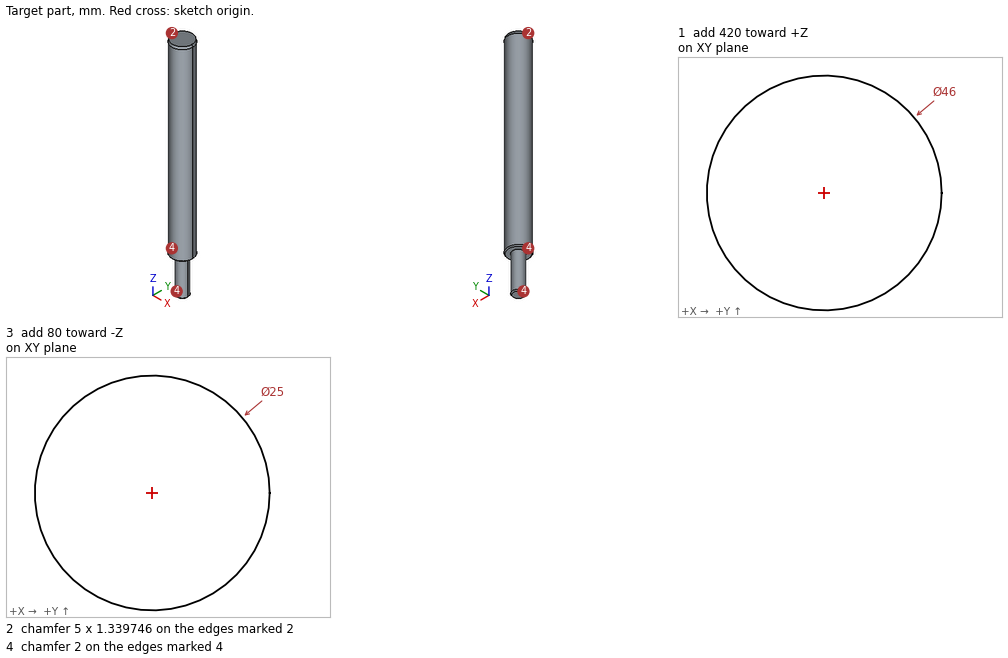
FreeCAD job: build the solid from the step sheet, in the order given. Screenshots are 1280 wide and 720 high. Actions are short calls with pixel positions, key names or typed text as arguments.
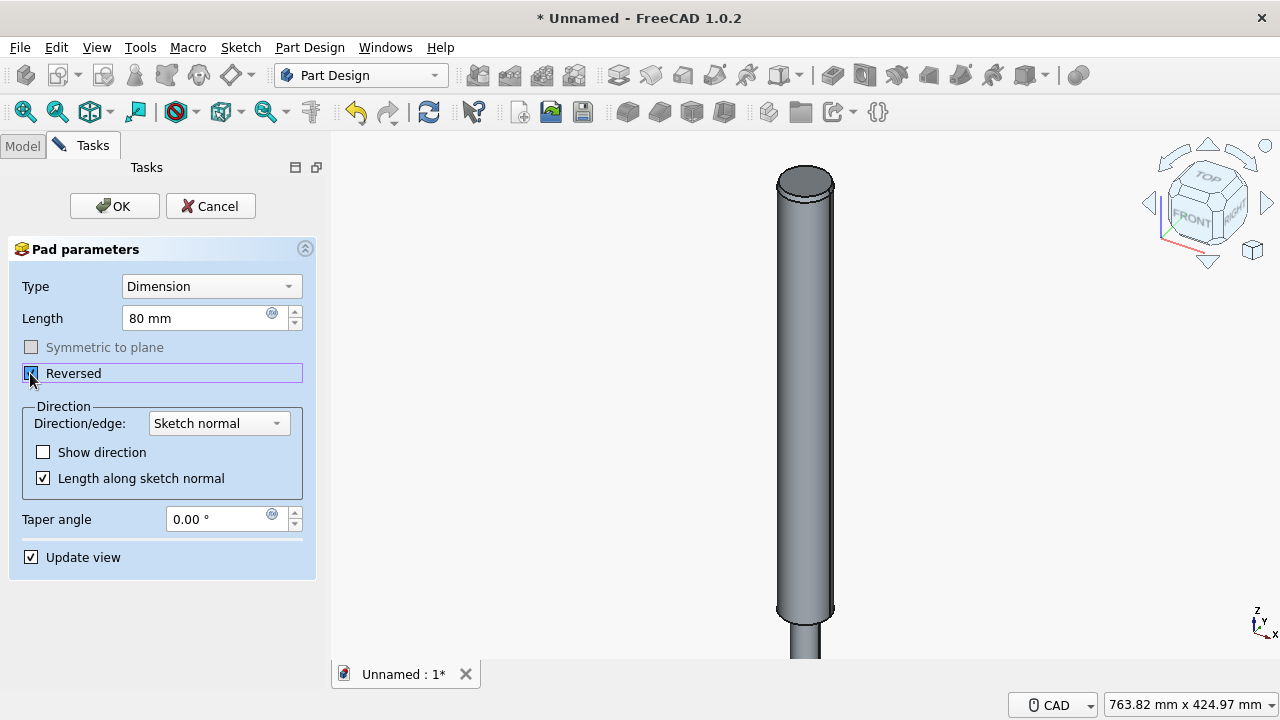
click(115, 206)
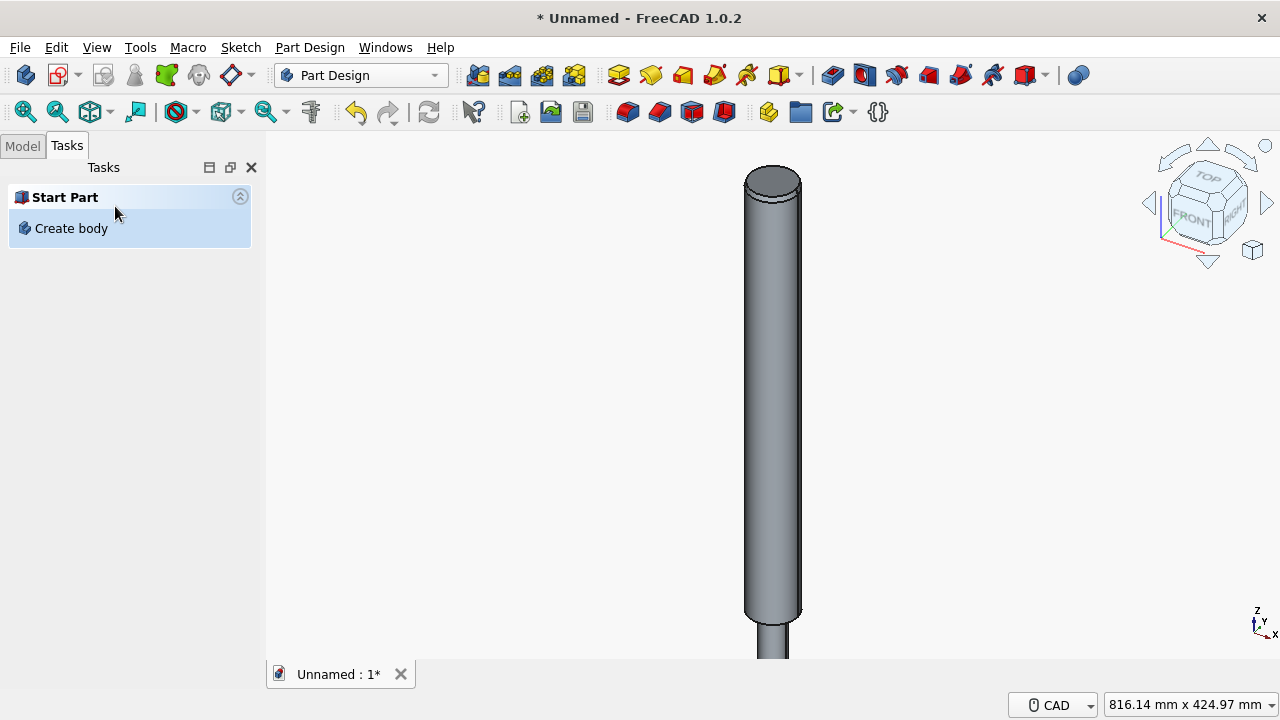
click(26, 112)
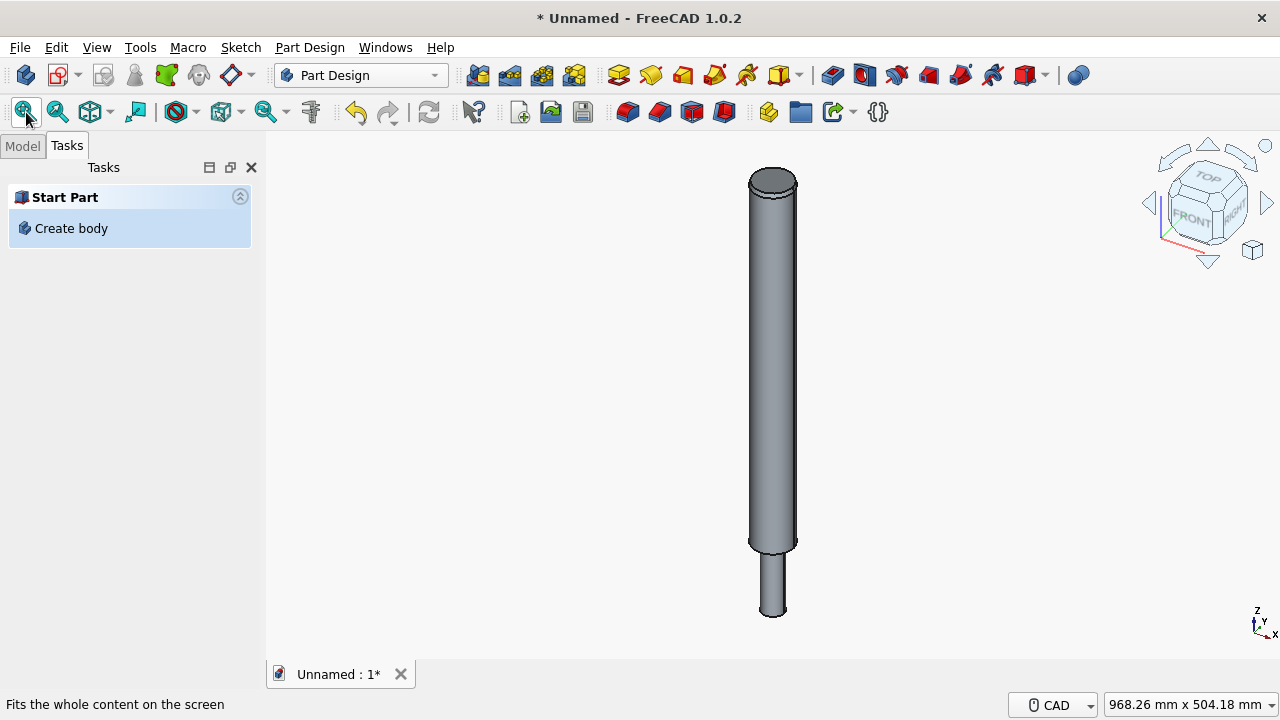
click(755, 549)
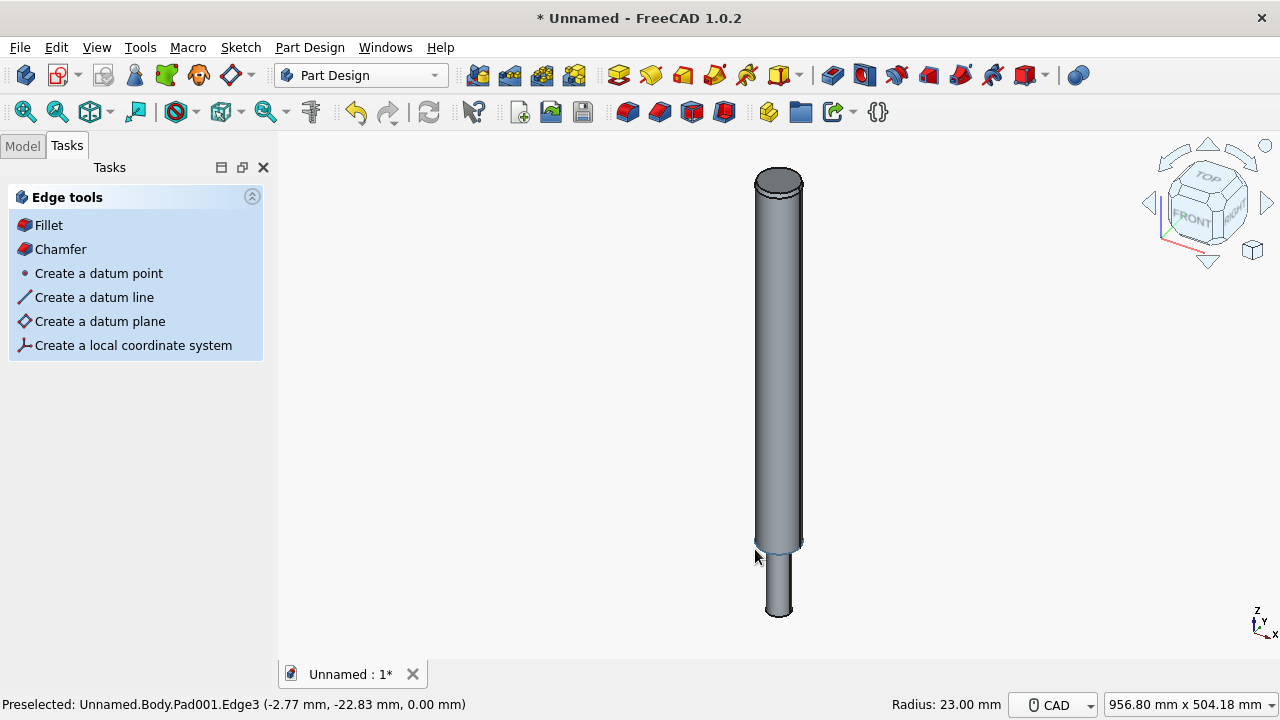
key(0)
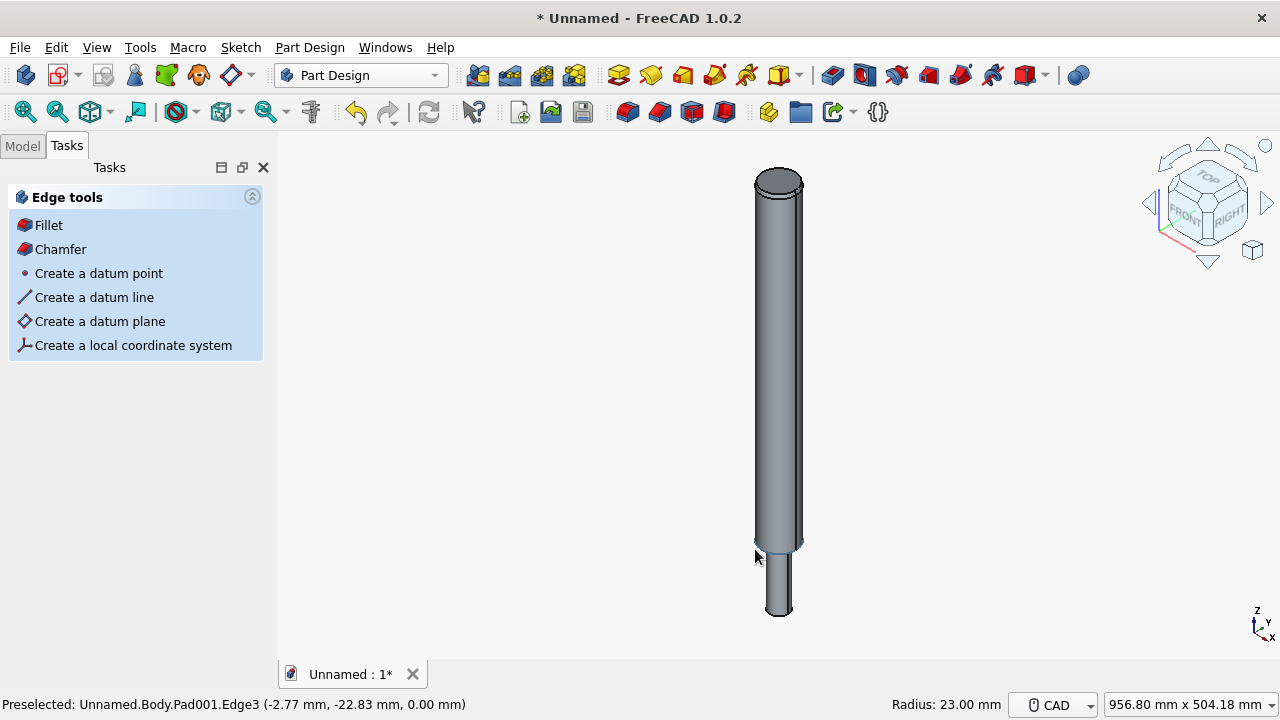
click(773, 615, ctrl)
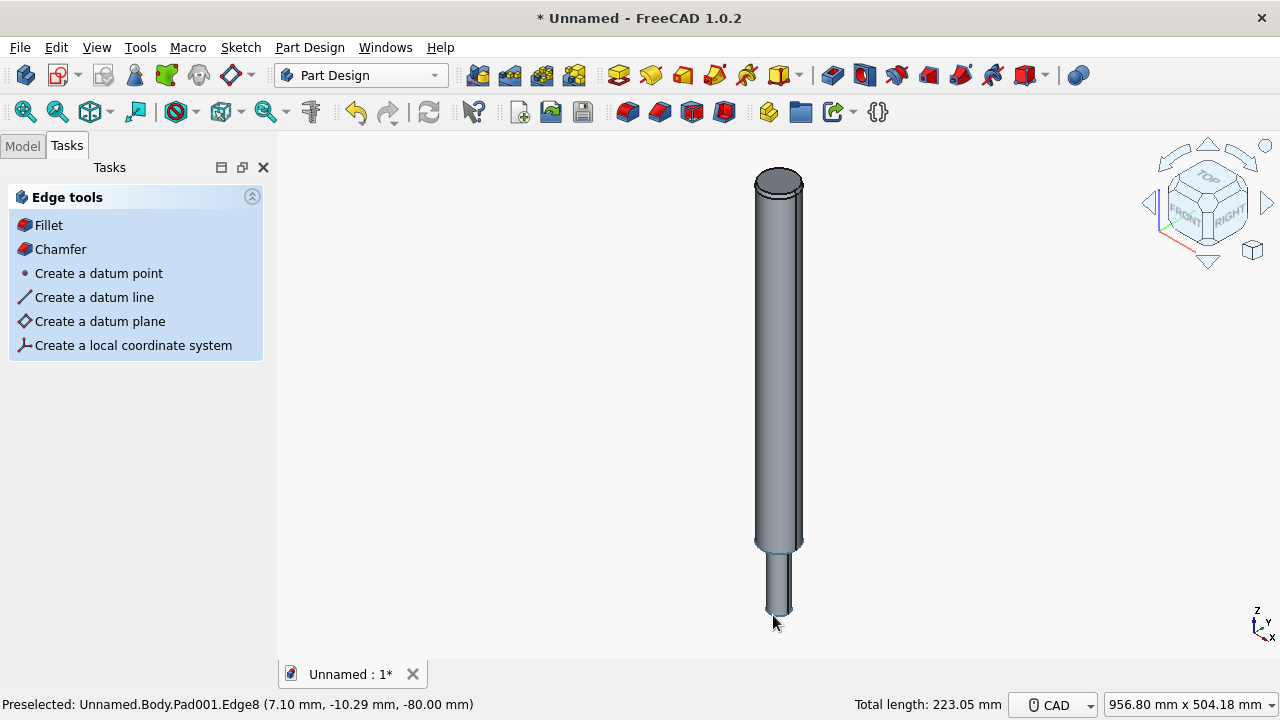
click(660, 112)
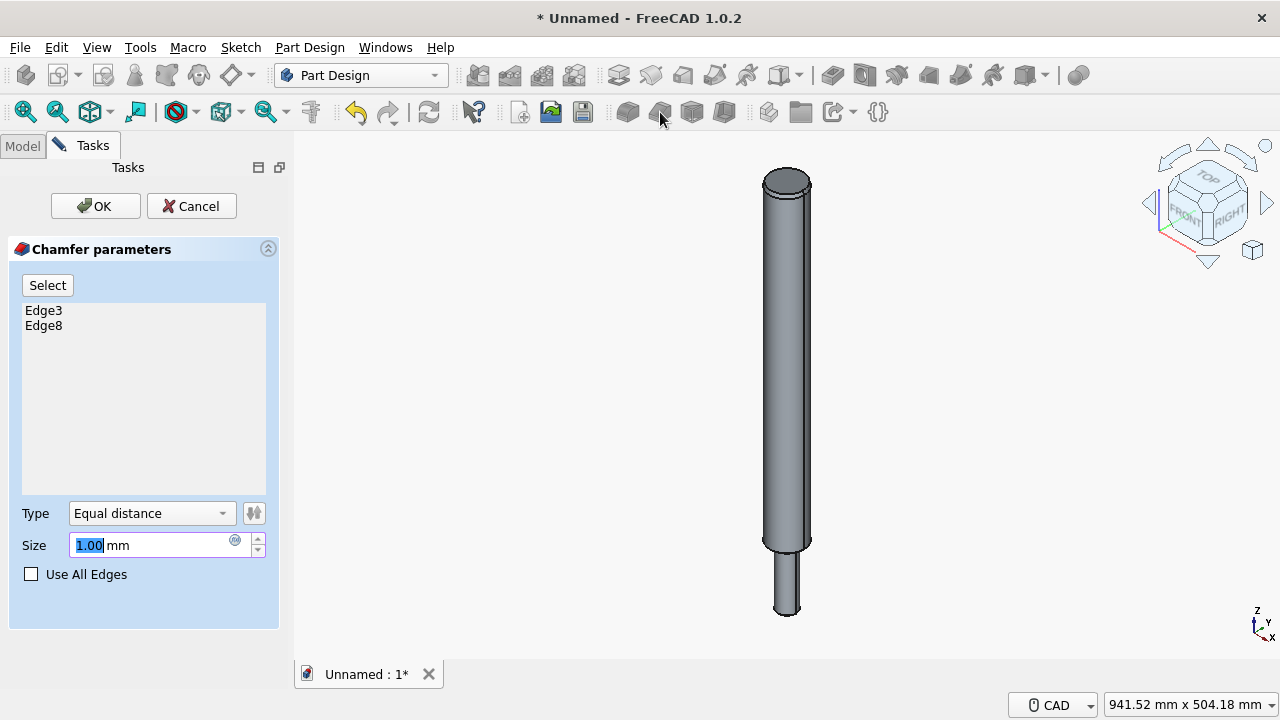
text(2)
key(Tab)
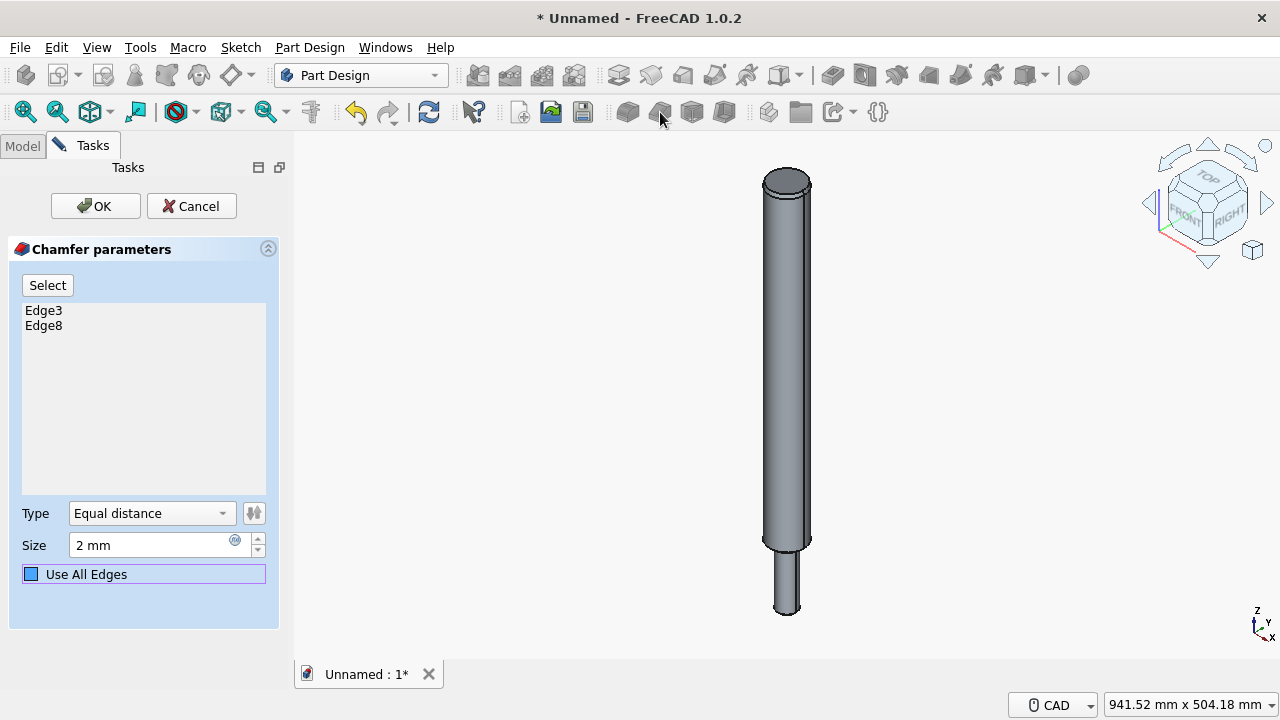
click(96, 206)